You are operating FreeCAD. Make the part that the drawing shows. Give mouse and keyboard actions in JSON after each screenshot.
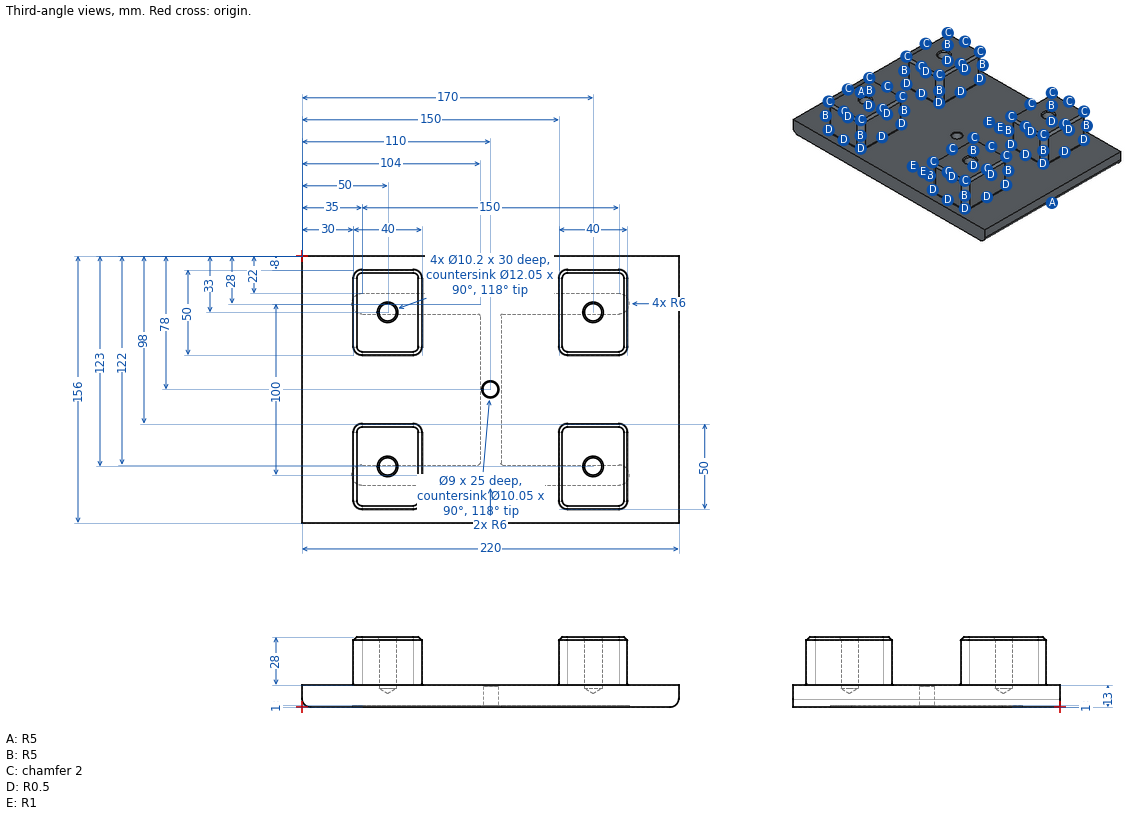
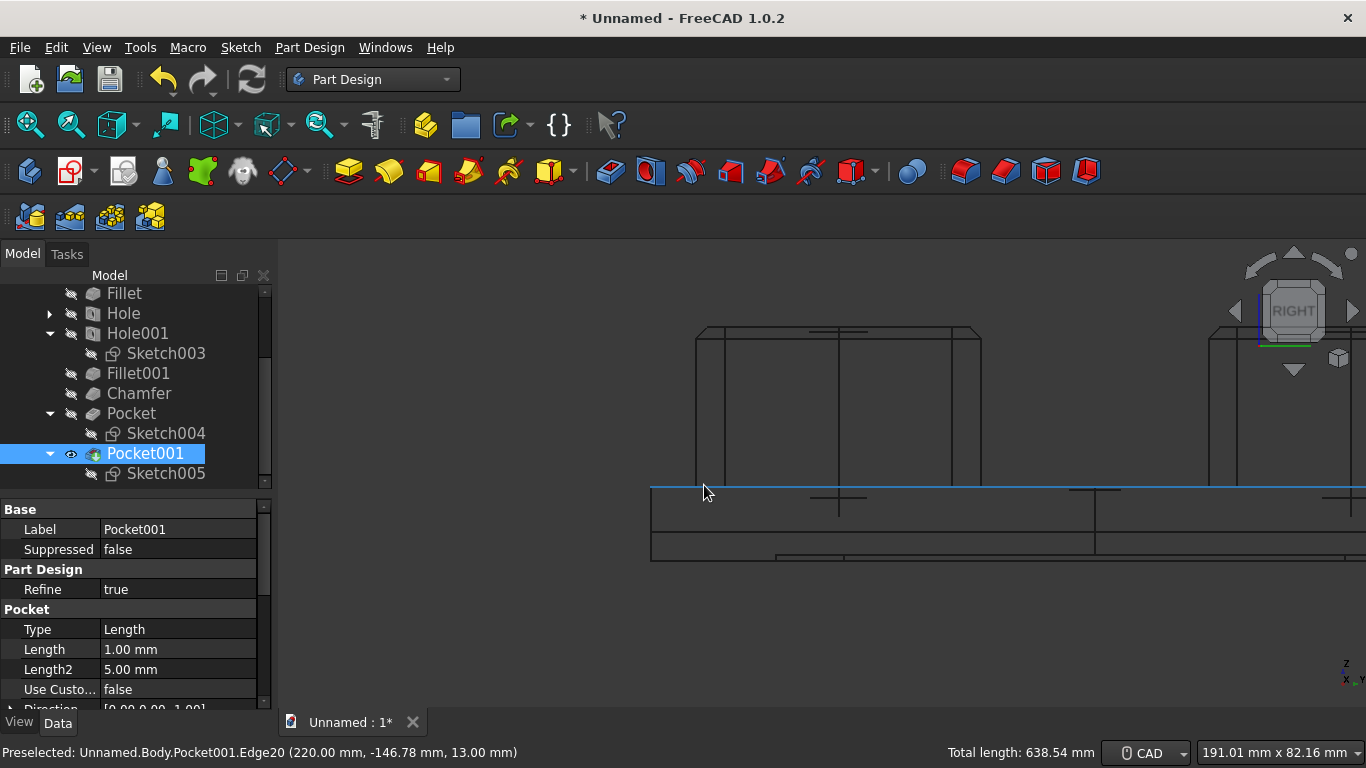
{"action": "key", "text": "v f"}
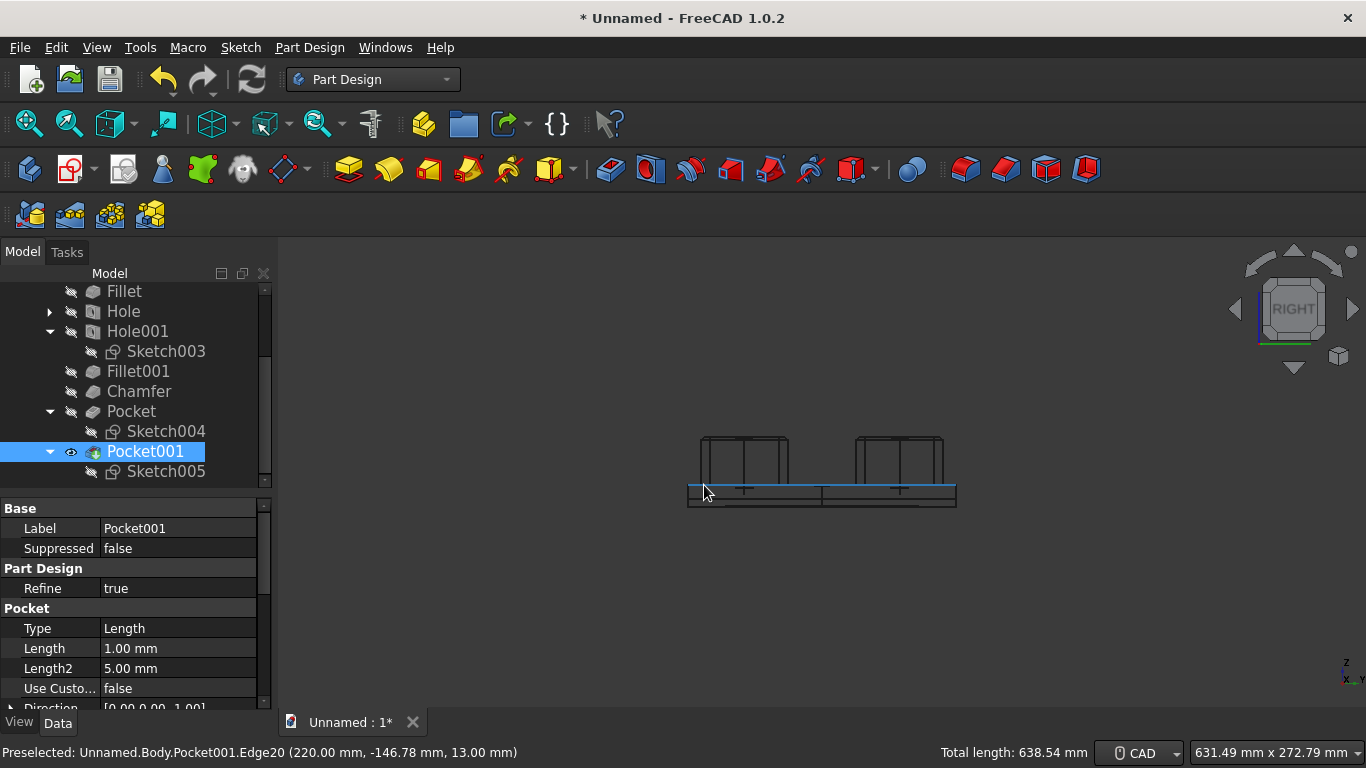
{"action": "key", "text": "5"}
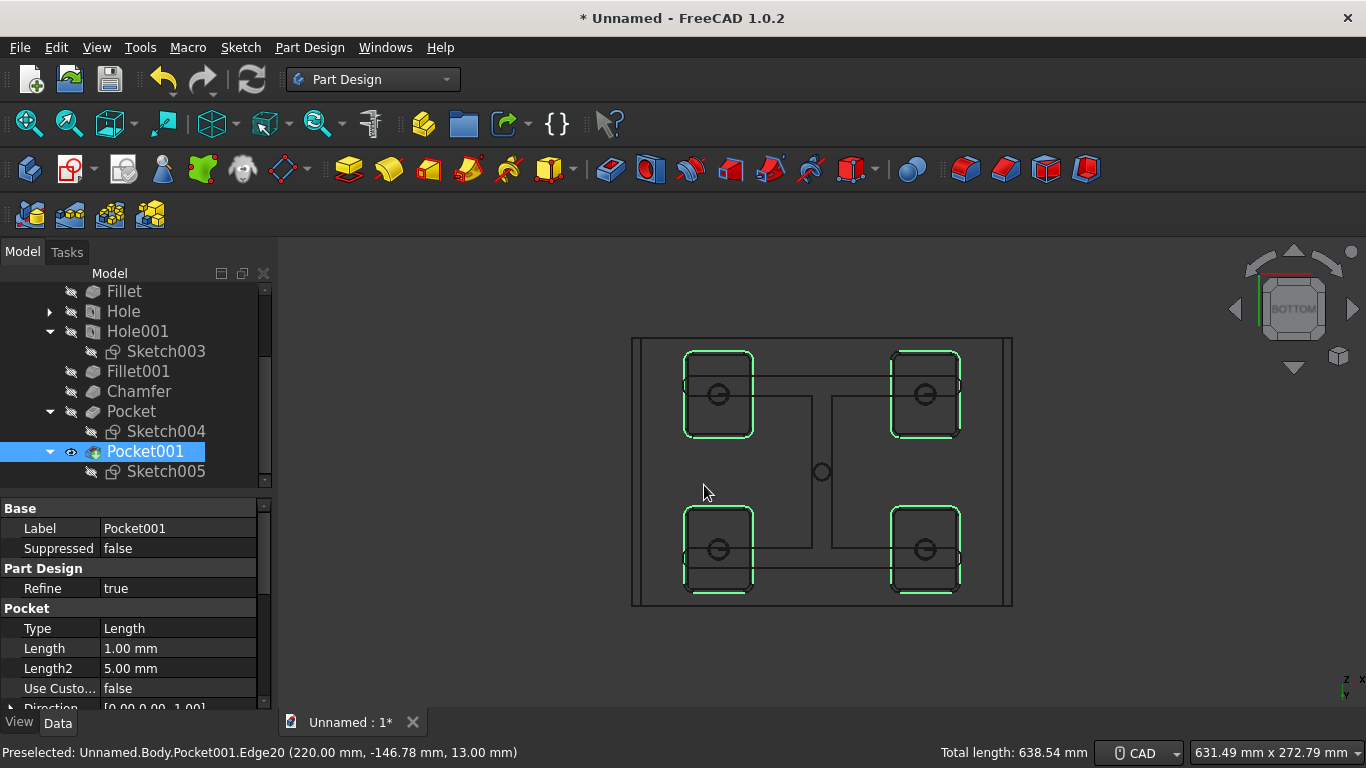
{"action": "left_click", "coordinate": [893, 353], "text": "ctrl"}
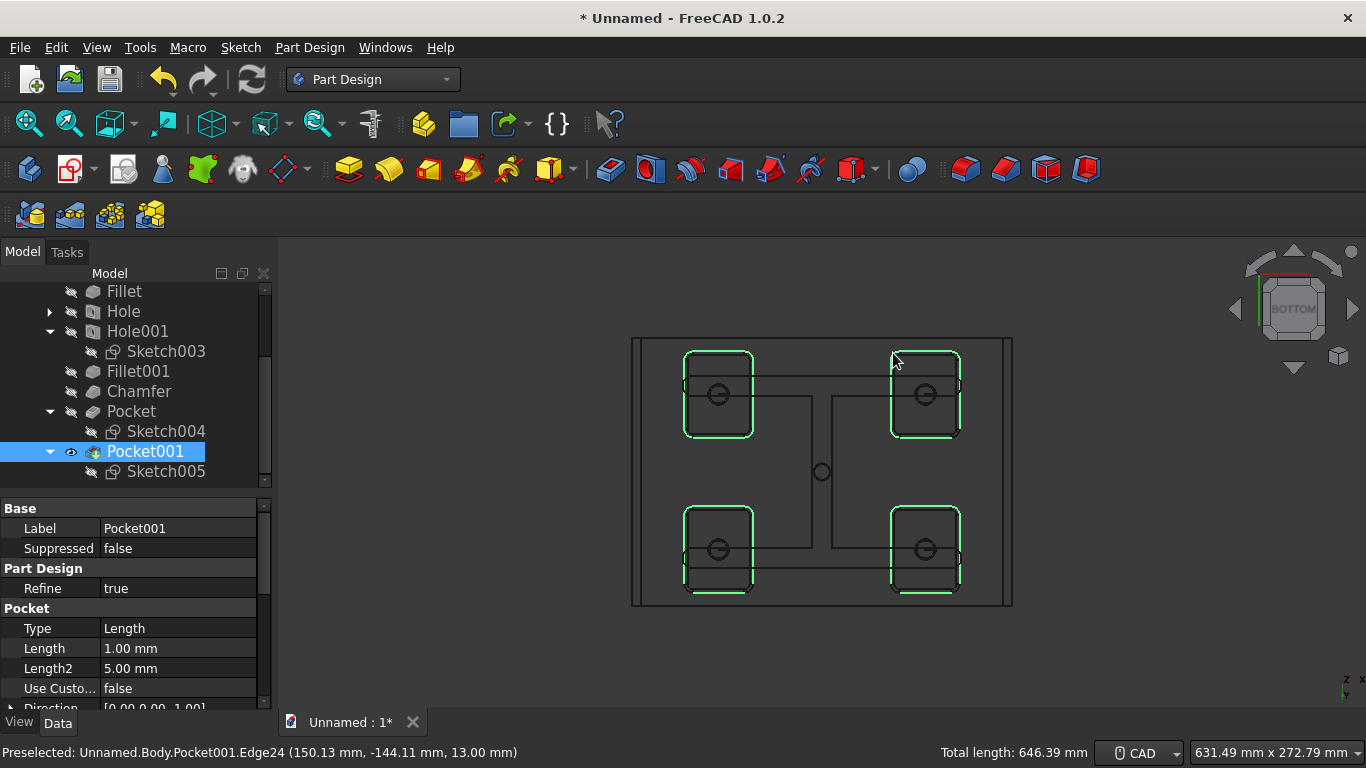
{"action": "left_click", "coordinate": [957, 434], "text": "ctrl"}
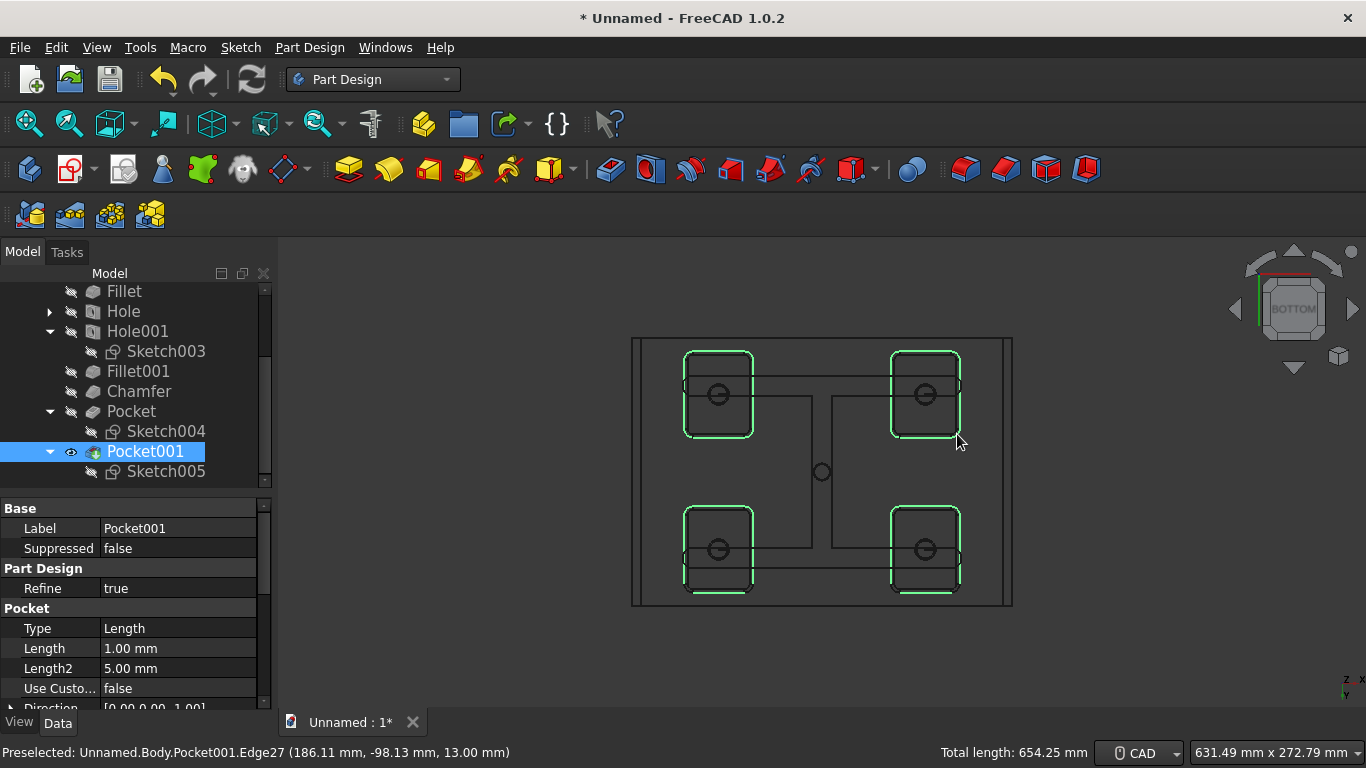
{"action": "left_click", "coordinate": [893, 589], "text": "ctrl"}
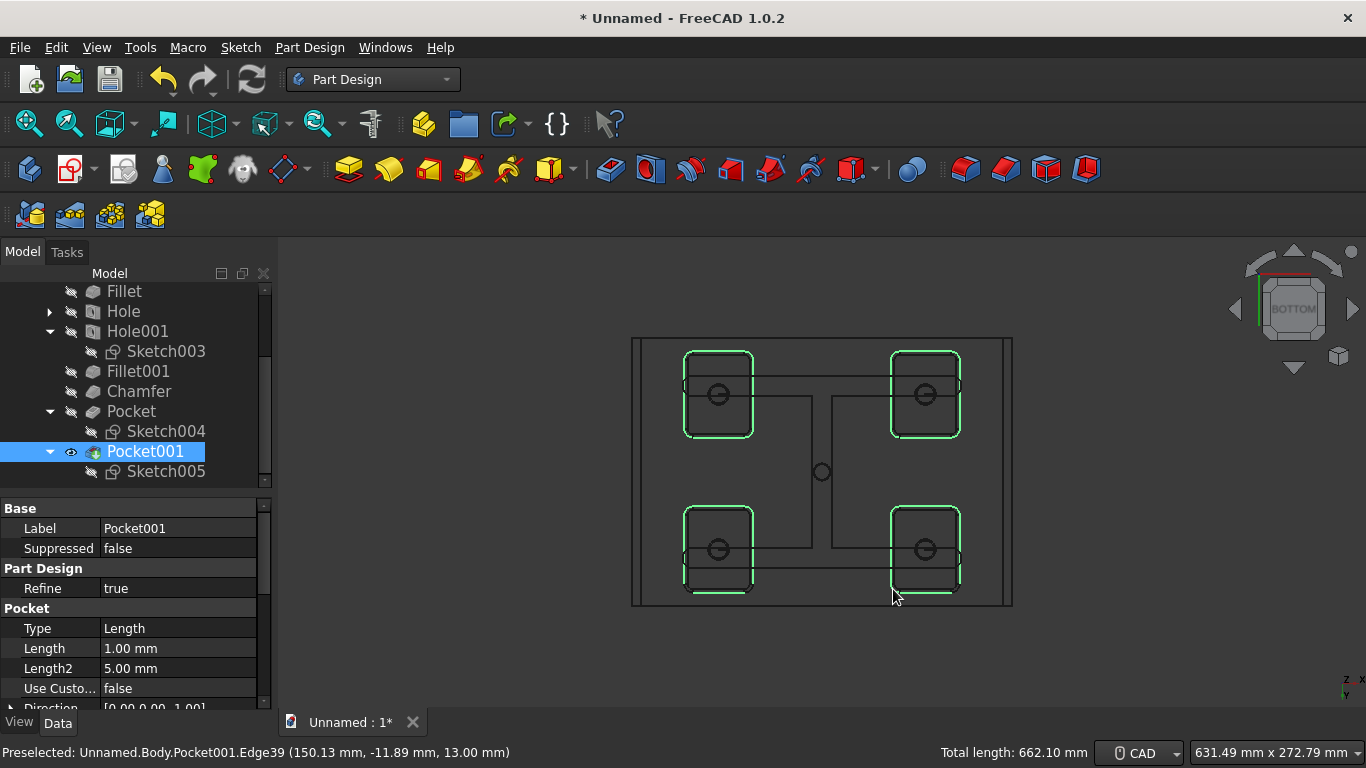
{"action": "left_click", "coordinate": [957, 589], "text": "ctrl"}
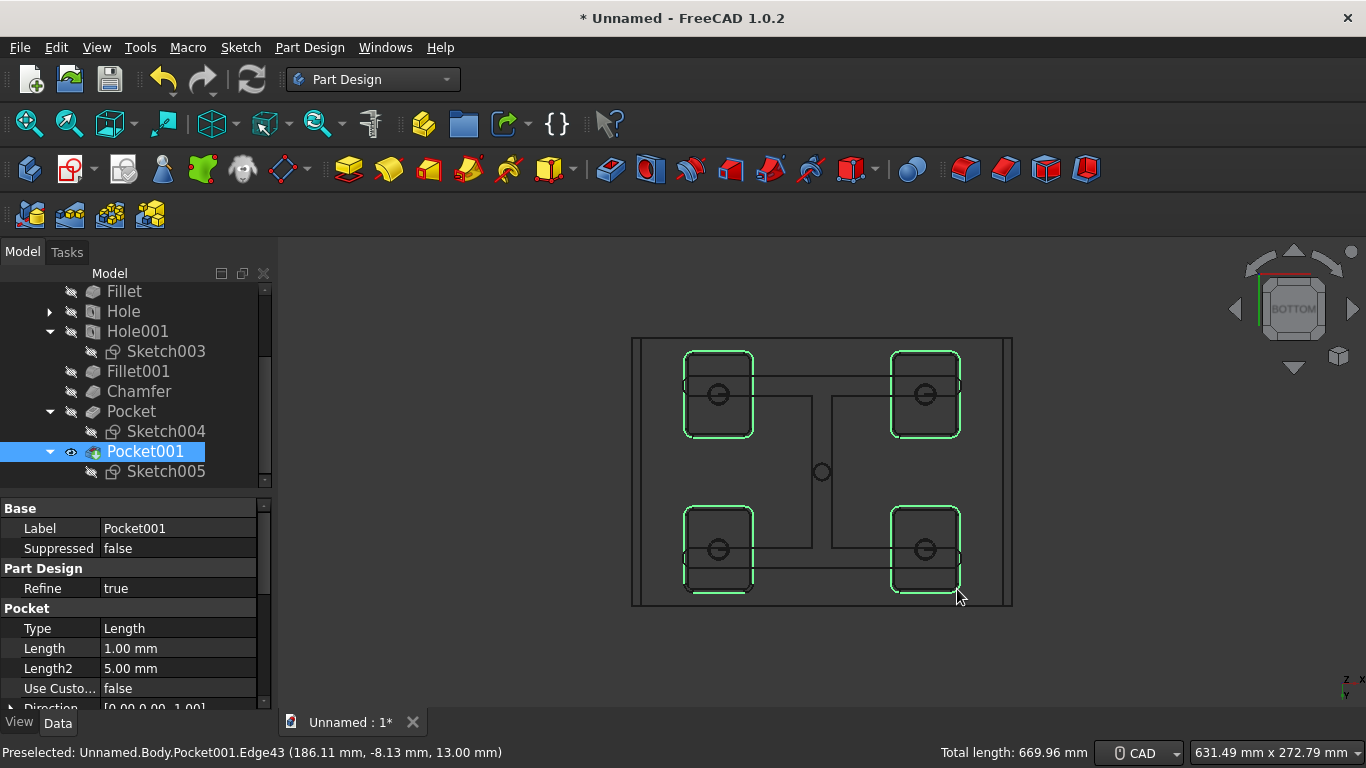
{"action": "left_click", "coordinate": [751, 589], "text": "ctrl"}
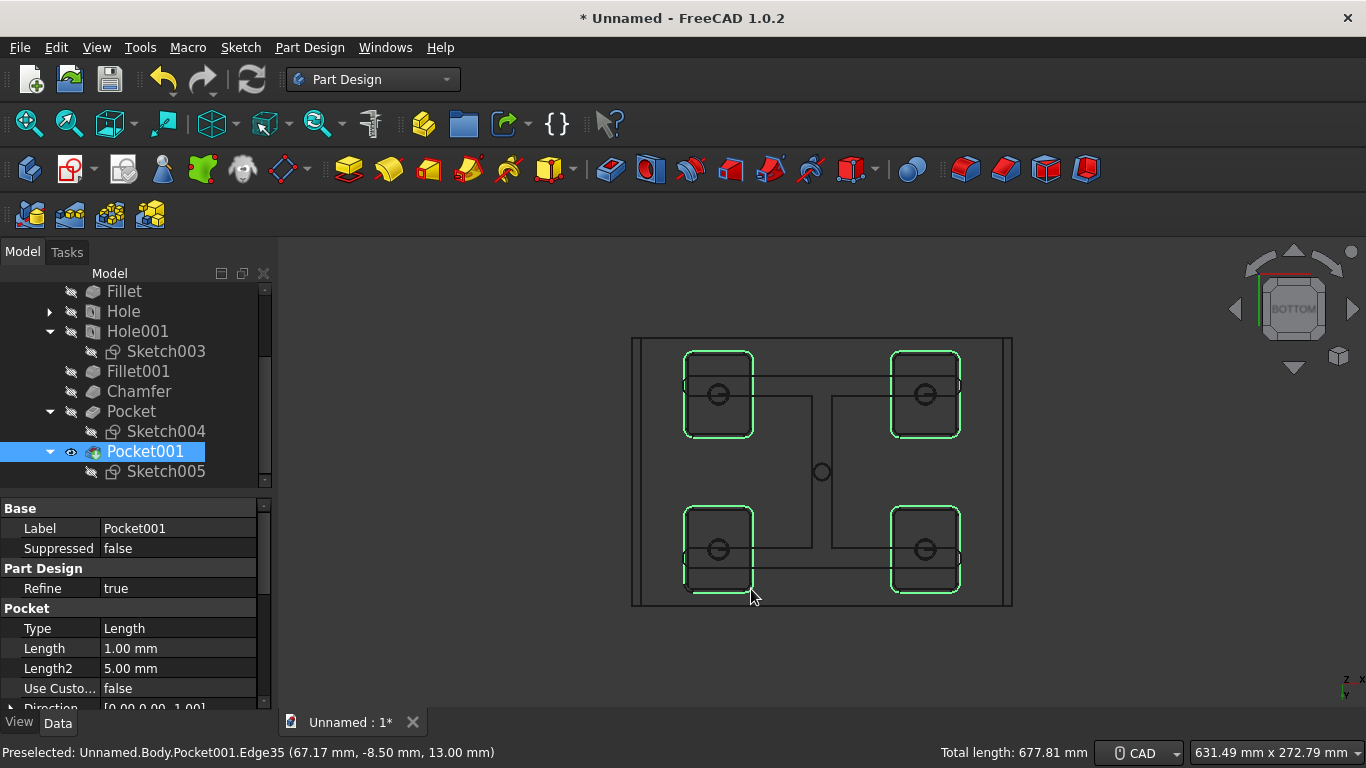
{"action": "left_click", "coordinate": [687, 589], "text": "ctrl"}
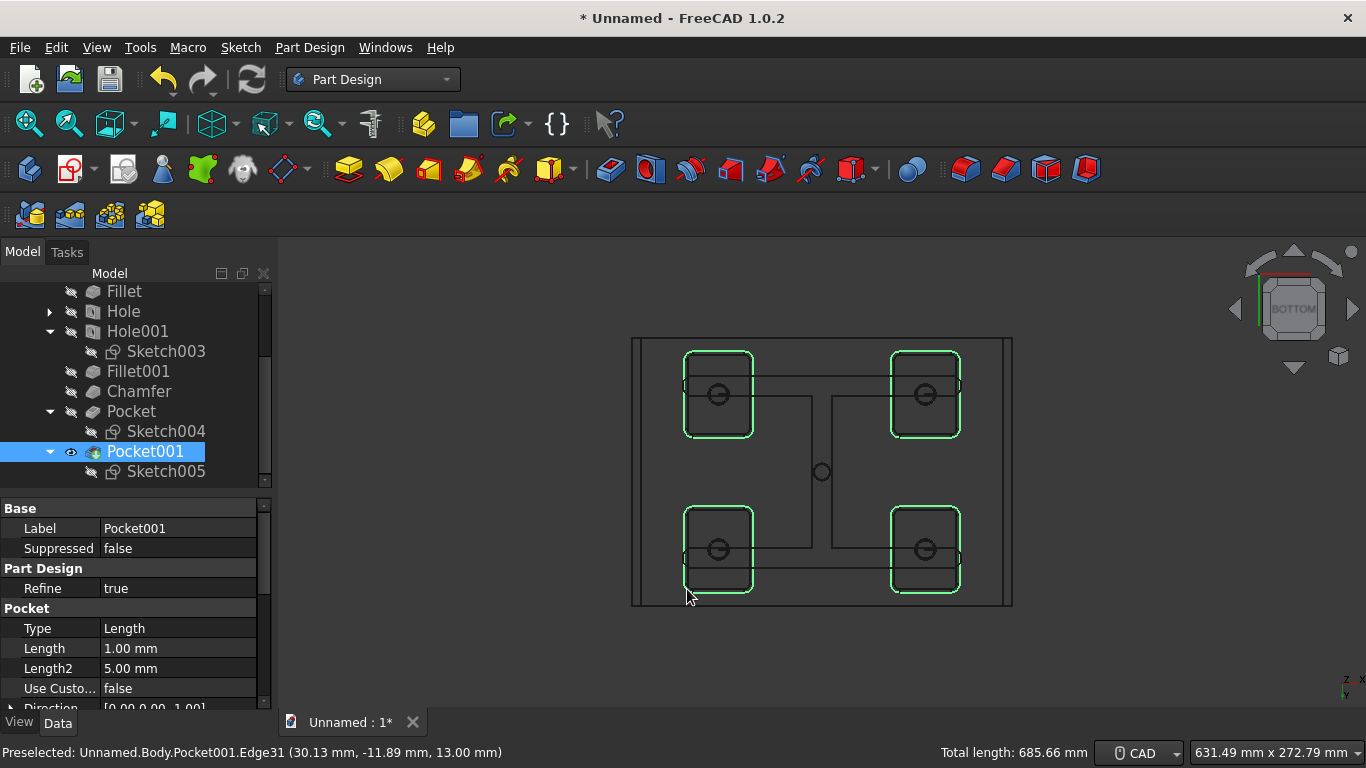
{"action": "key", "text": "v 1"}